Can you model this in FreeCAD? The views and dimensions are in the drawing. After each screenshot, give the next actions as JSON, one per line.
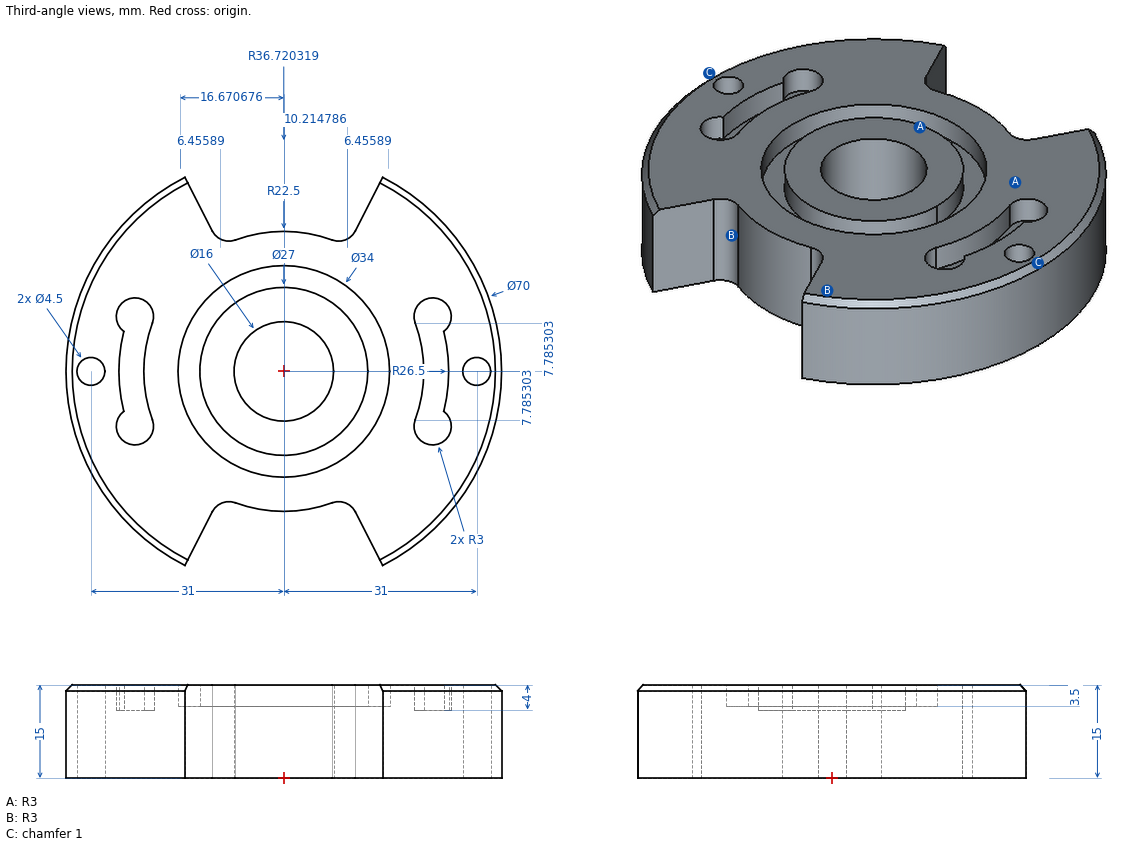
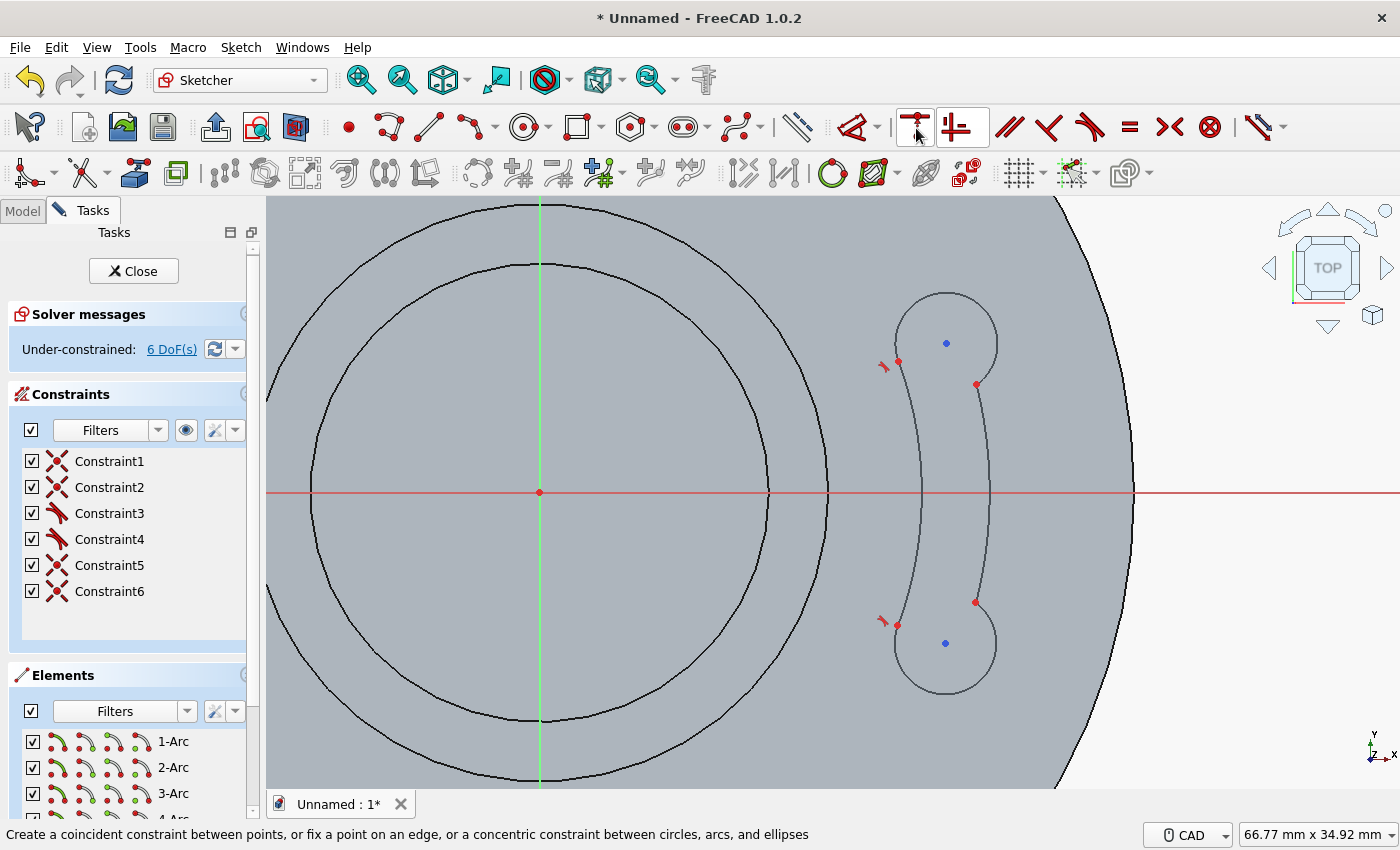
{"action": "left_click", "coordinate": [917, 686]}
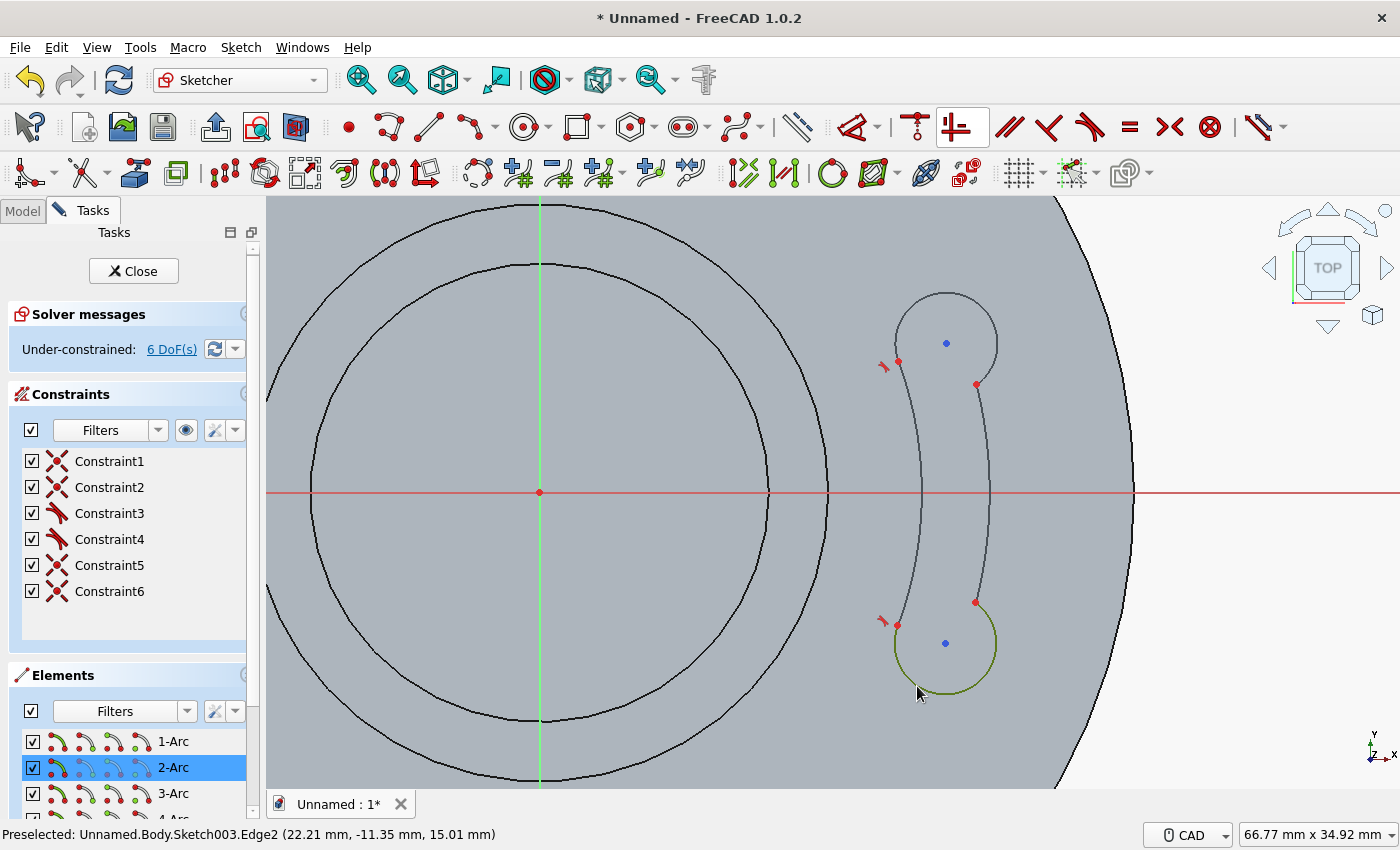
{"action": "left_click", "coordinate": [994, 324]}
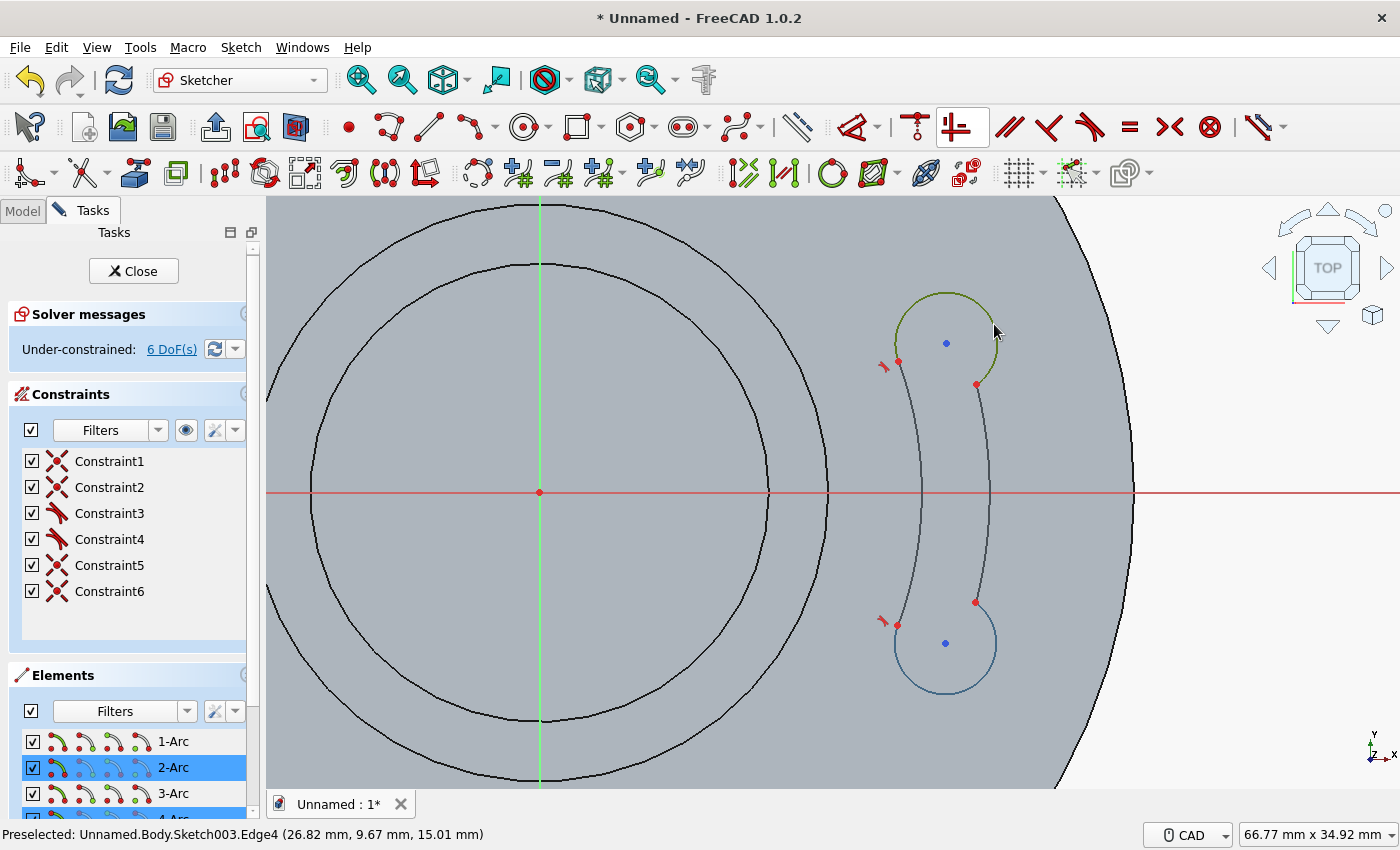
{"action": "left_click", "coordinate": [1130, 128]}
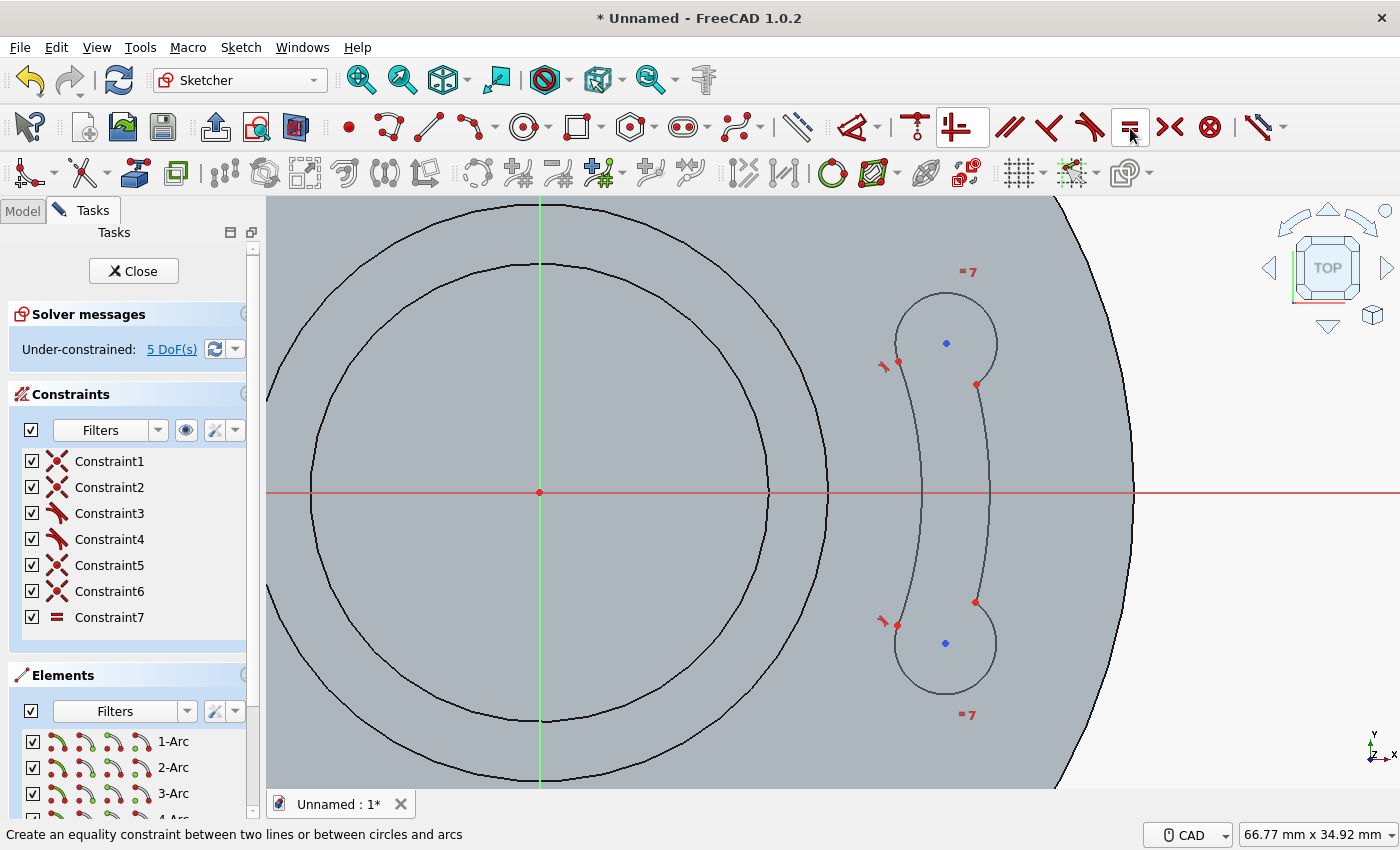
{"action": "left_click", "coordinate": [852, 128]}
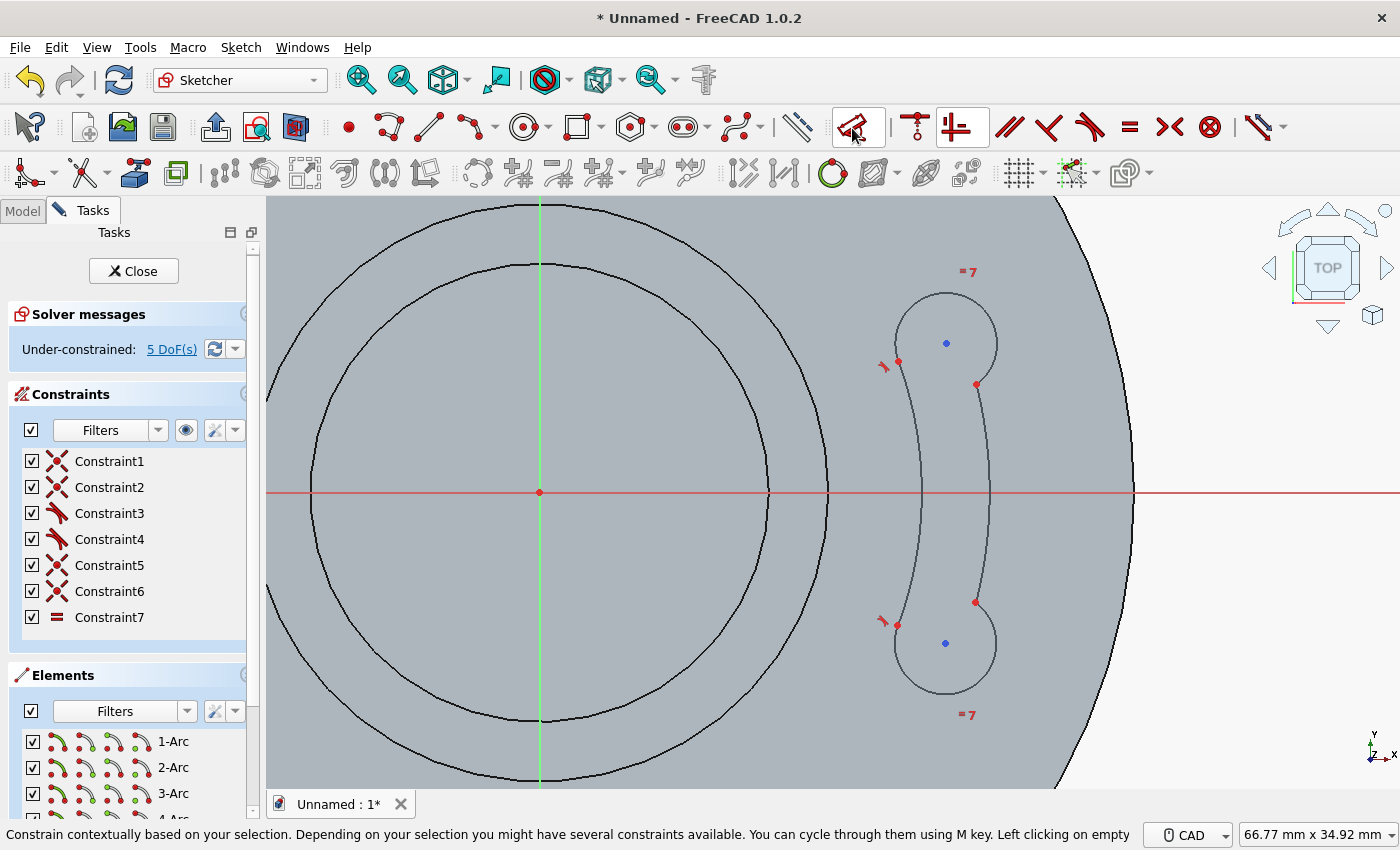
{"action": "left_click", "coordinate": [918, 548]}
{"action": "left_click", "coordinate": [950, 553]}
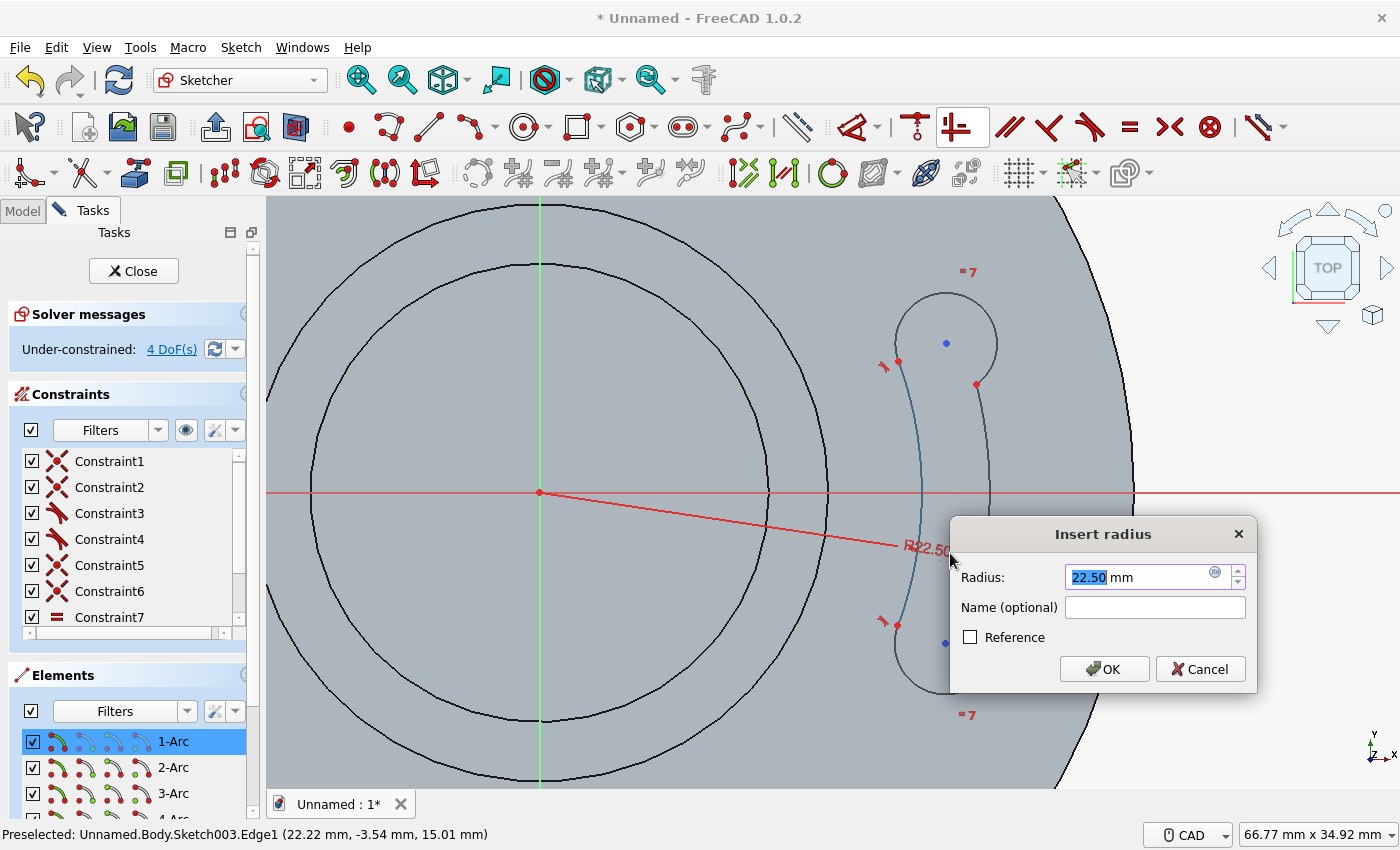
{"action": "type", "text": "22.5"}
{"action": "key", "text": "Return"}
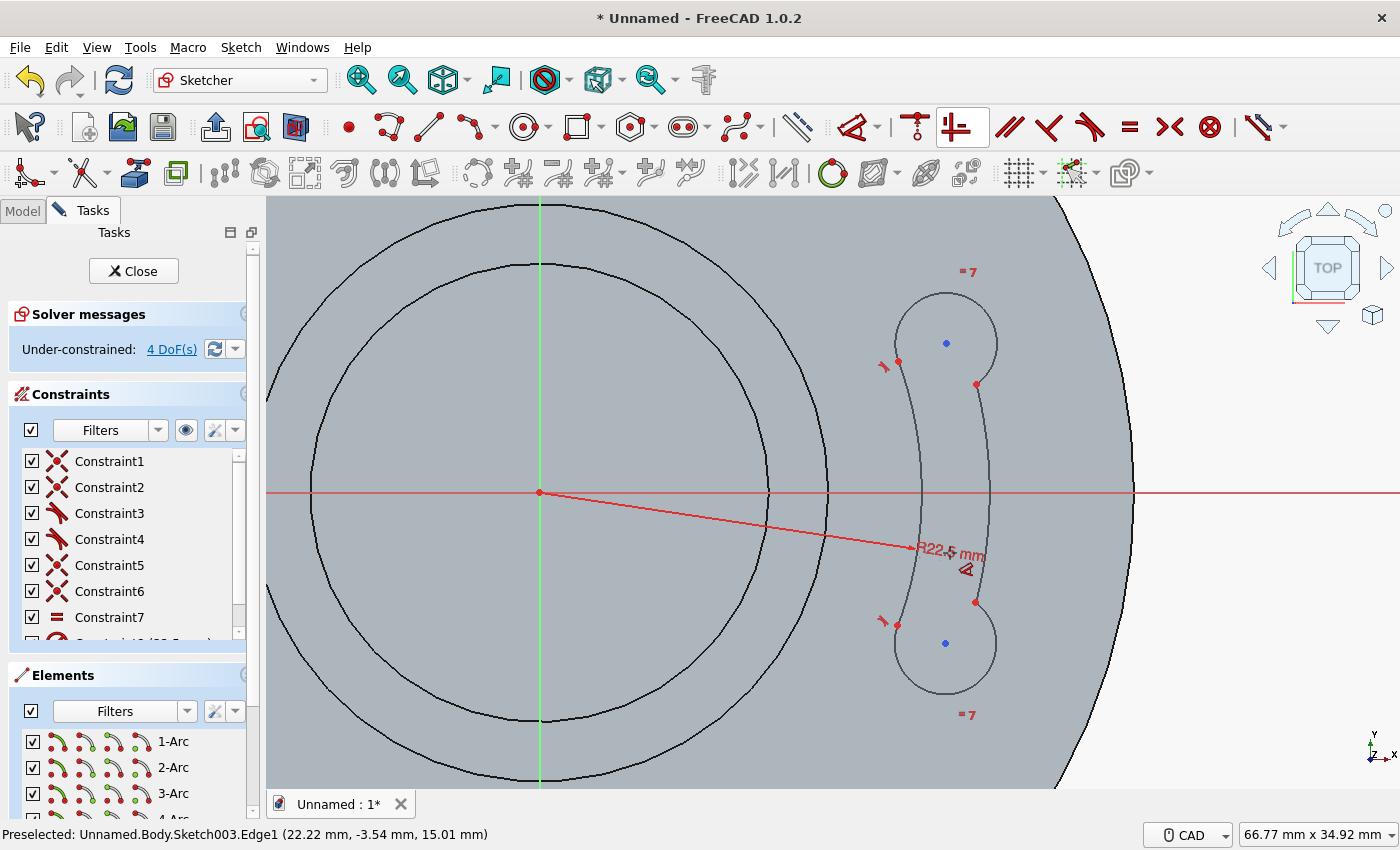
{"action": "left_click", "coordinate": [917, 686]}
{"action": "left_click", "coordinate": [899, 713]}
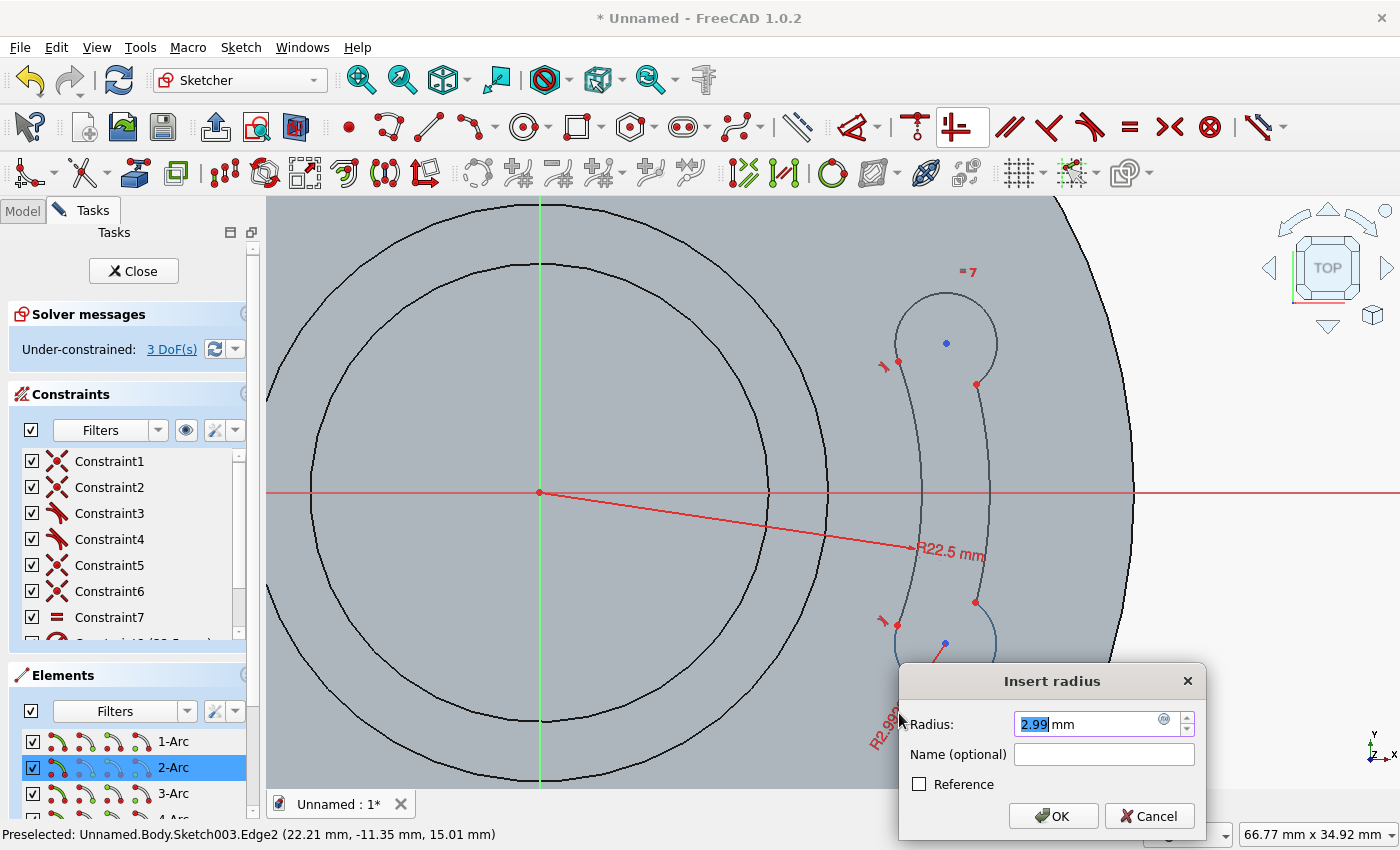
{"action": "type", "text": "3"}
{"action": "key", "text": "Return"}